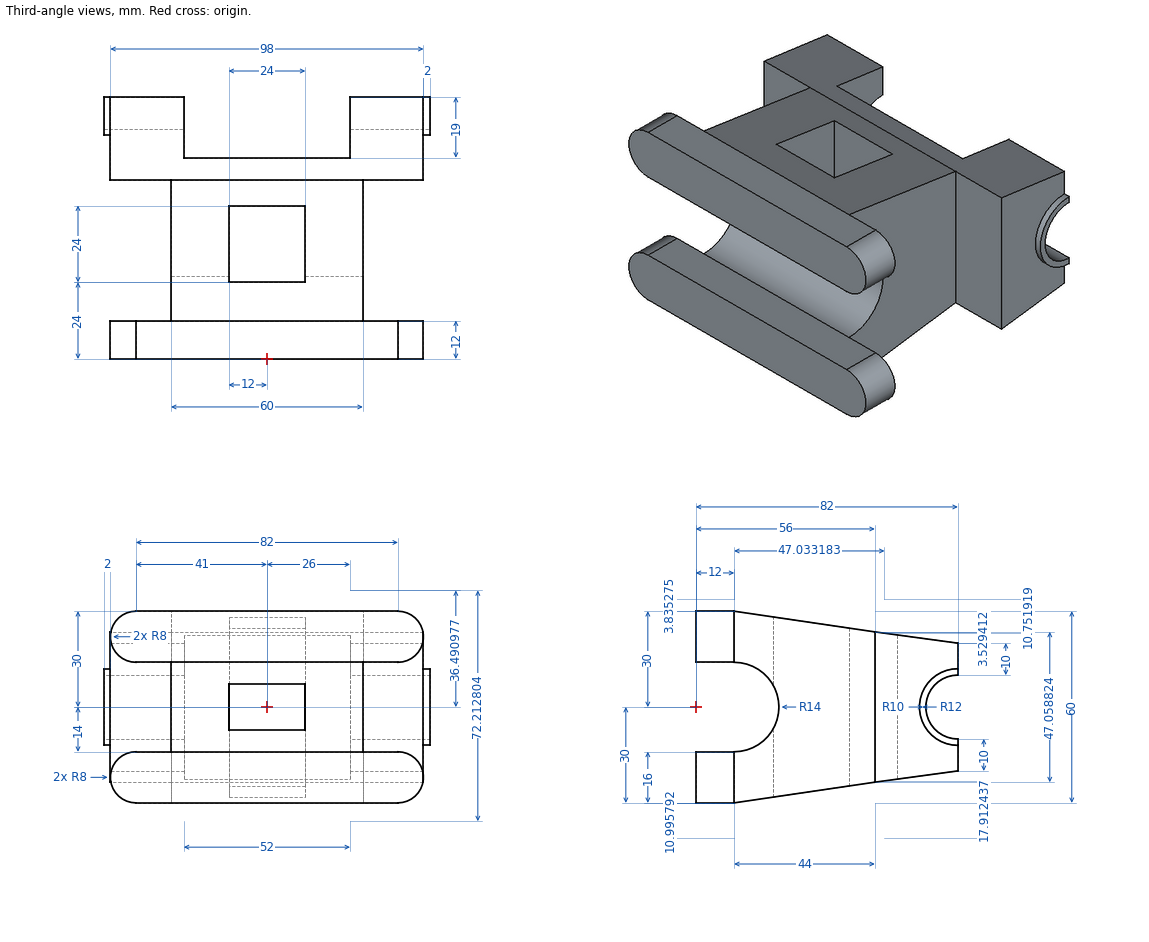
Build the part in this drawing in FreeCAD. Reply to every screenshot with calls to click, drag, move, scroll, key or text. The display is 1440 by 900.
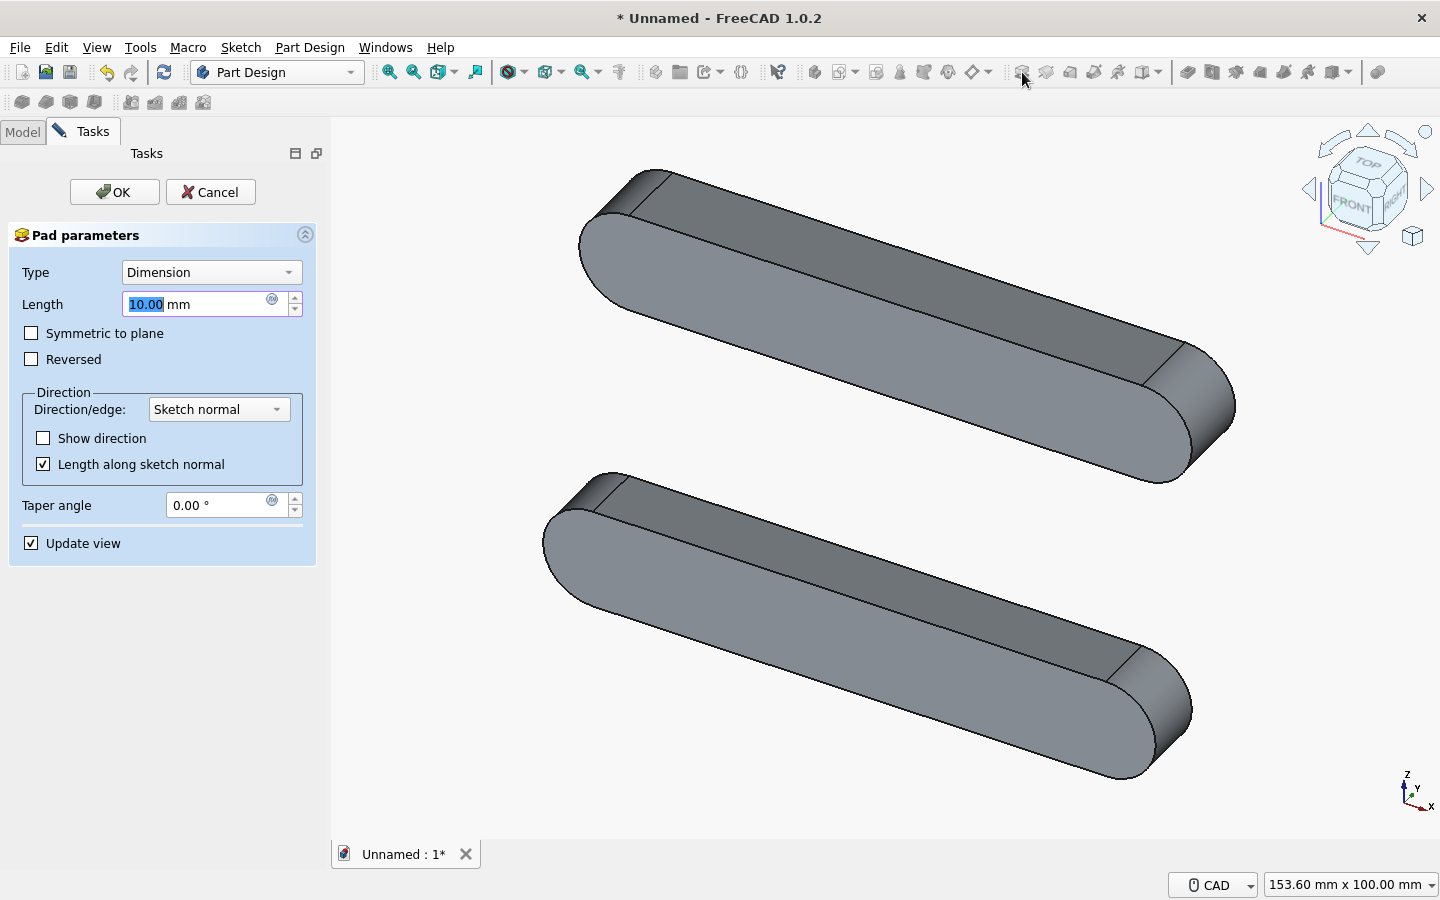
text(12)
key(Tab)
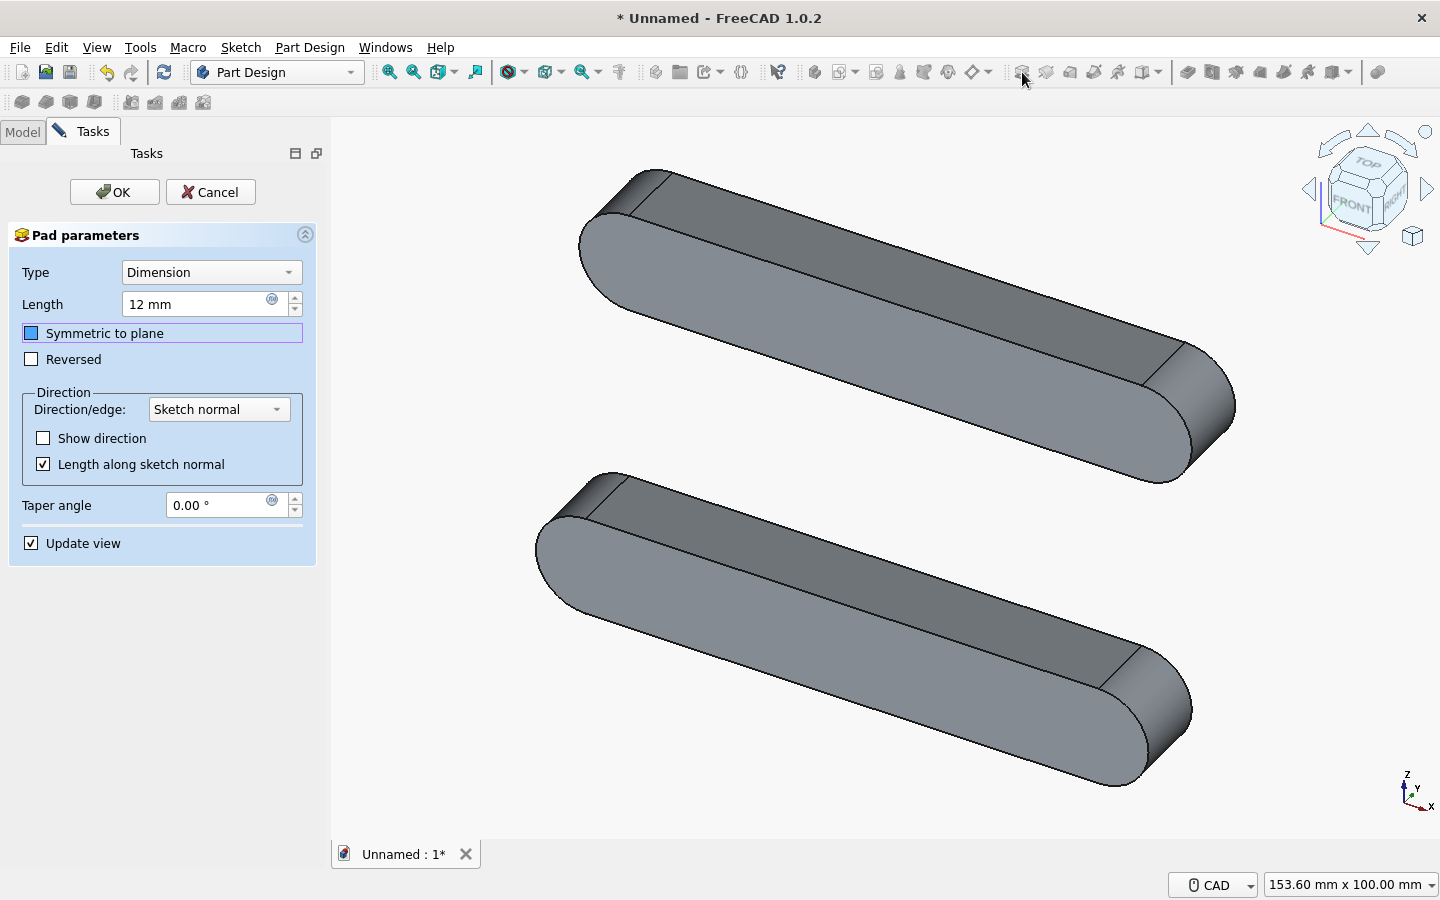
click(30, 359)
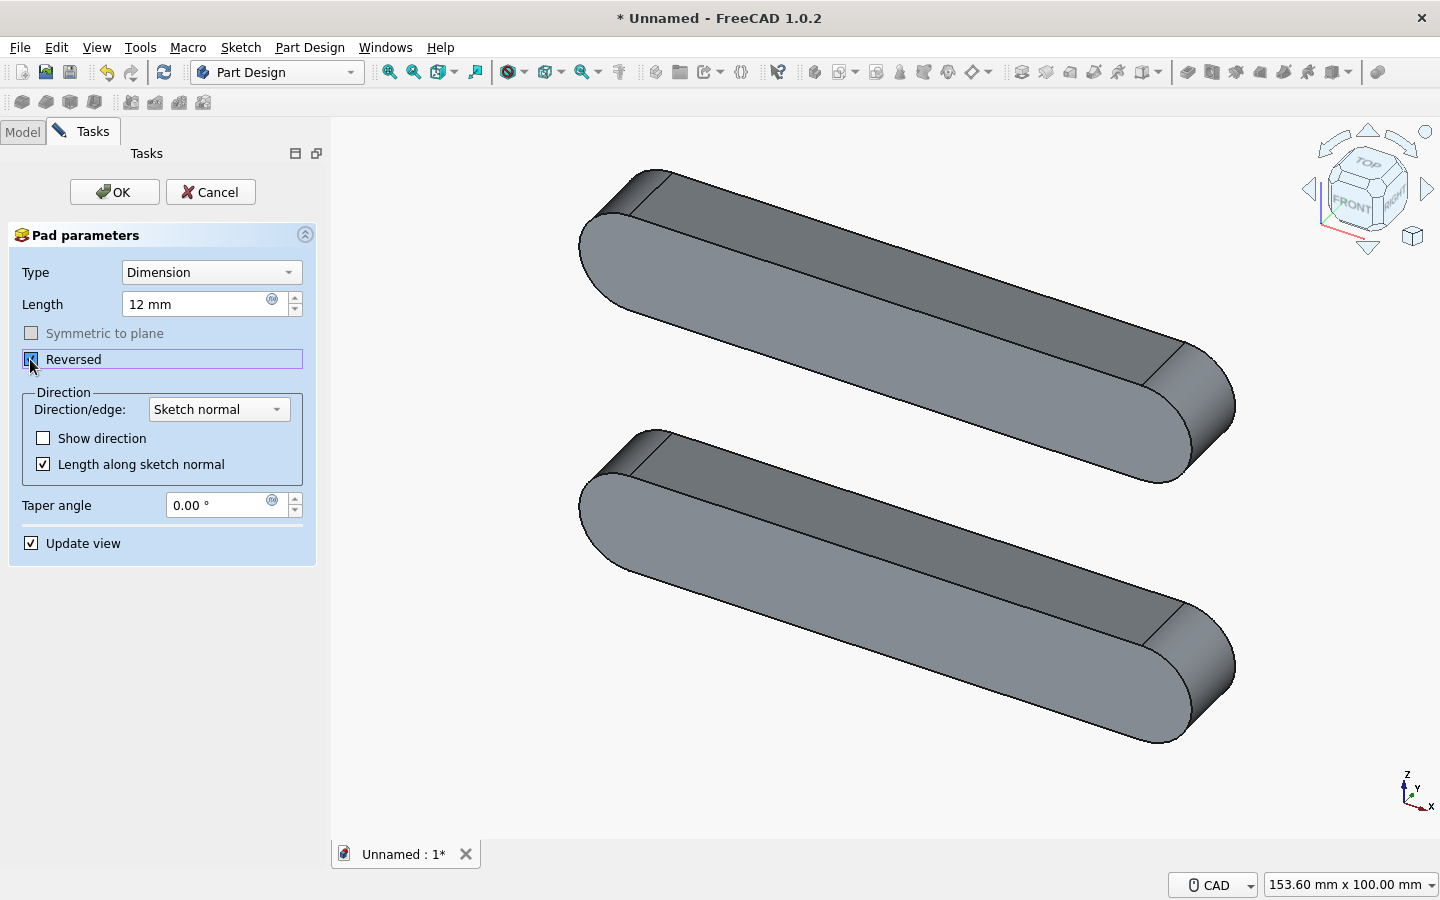
click(115, 192)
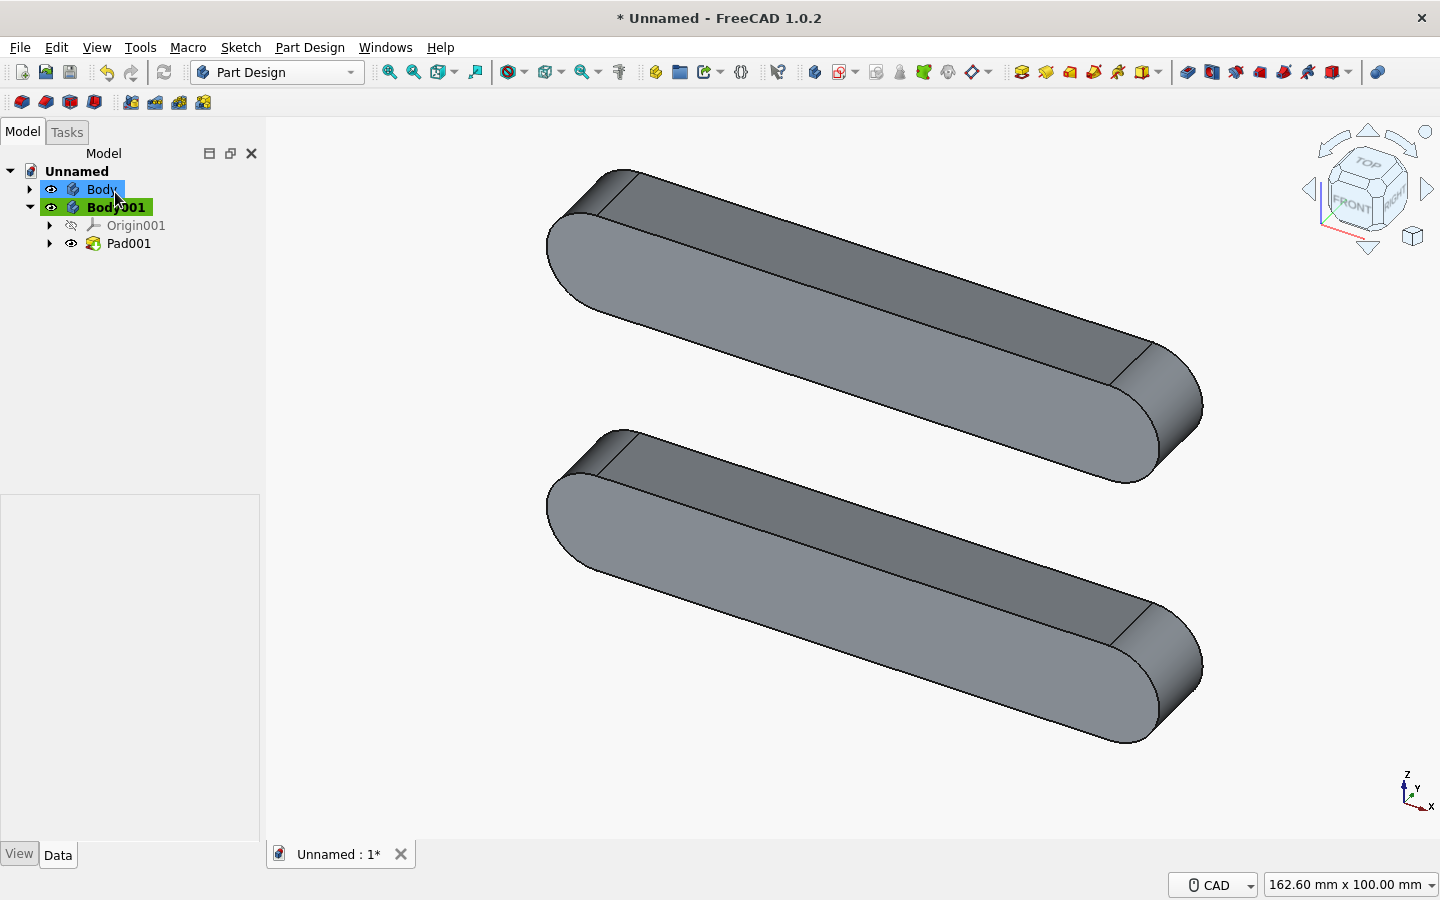
double_click(96, 189)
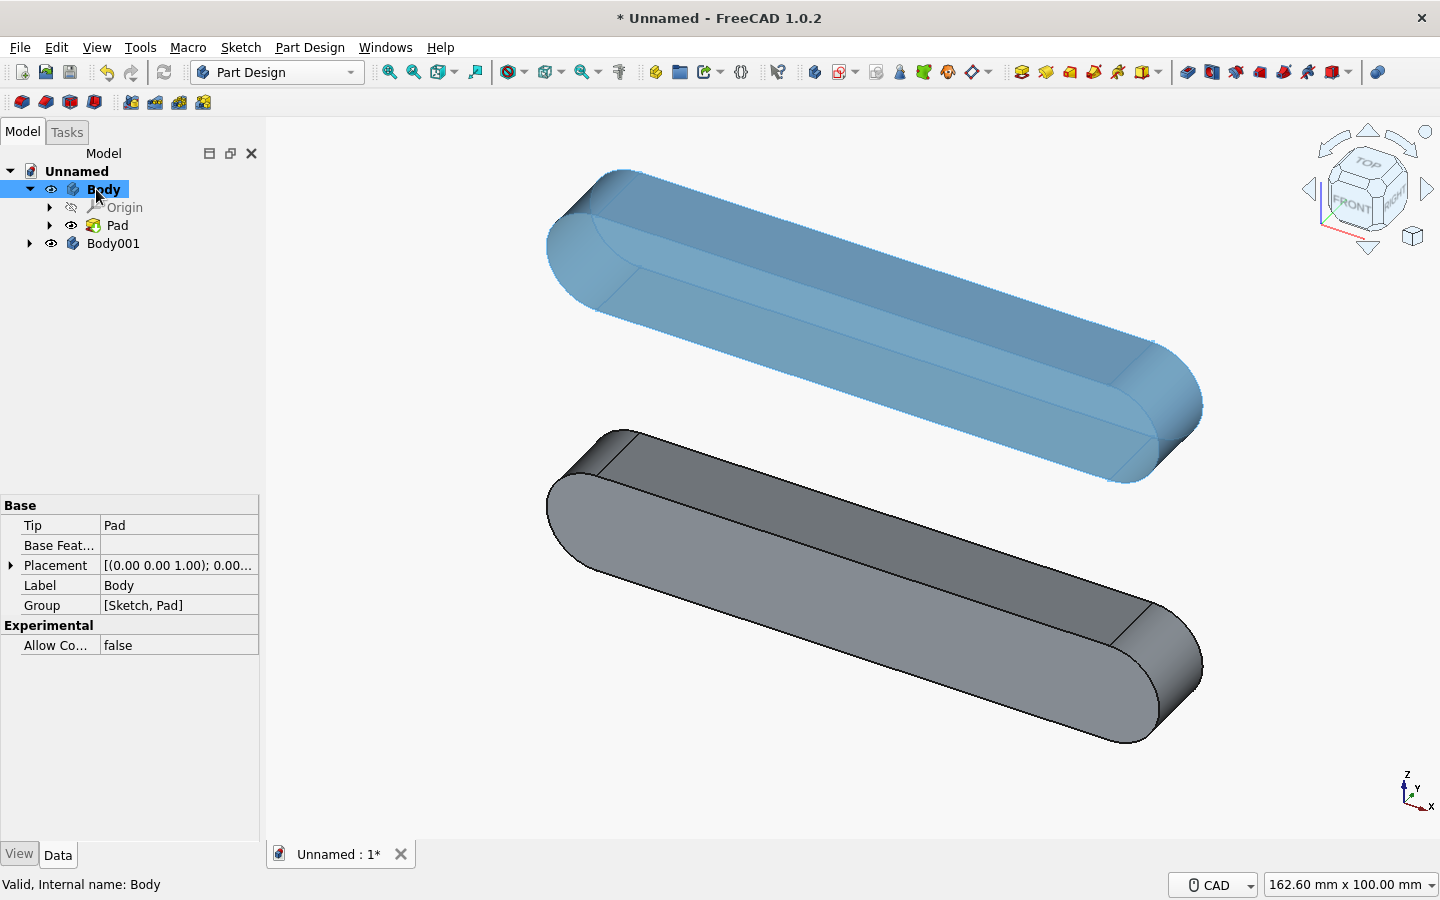
click(96, 189)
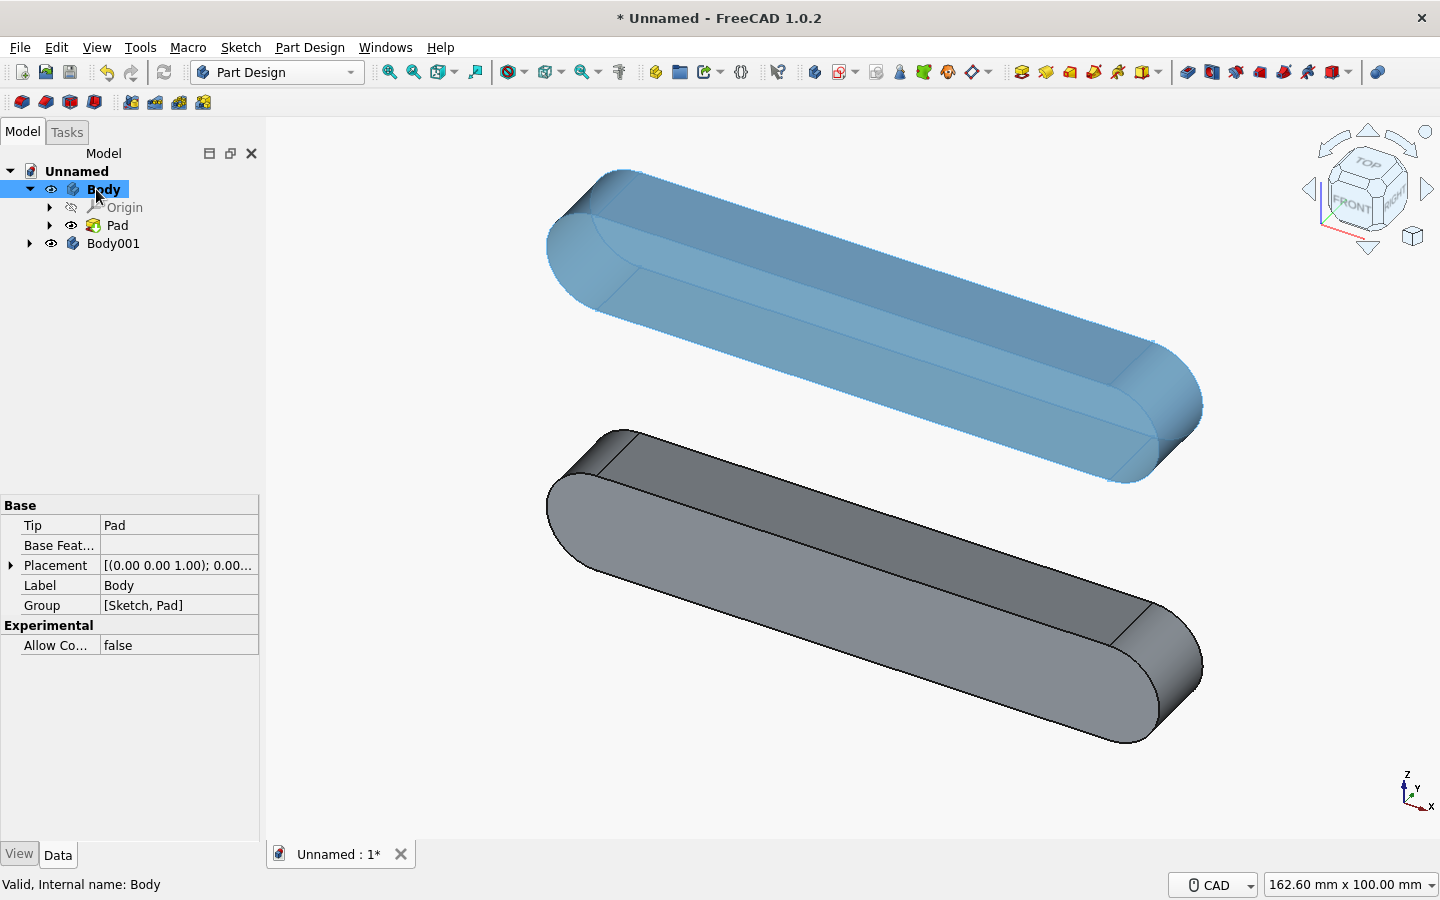
click(146, 645)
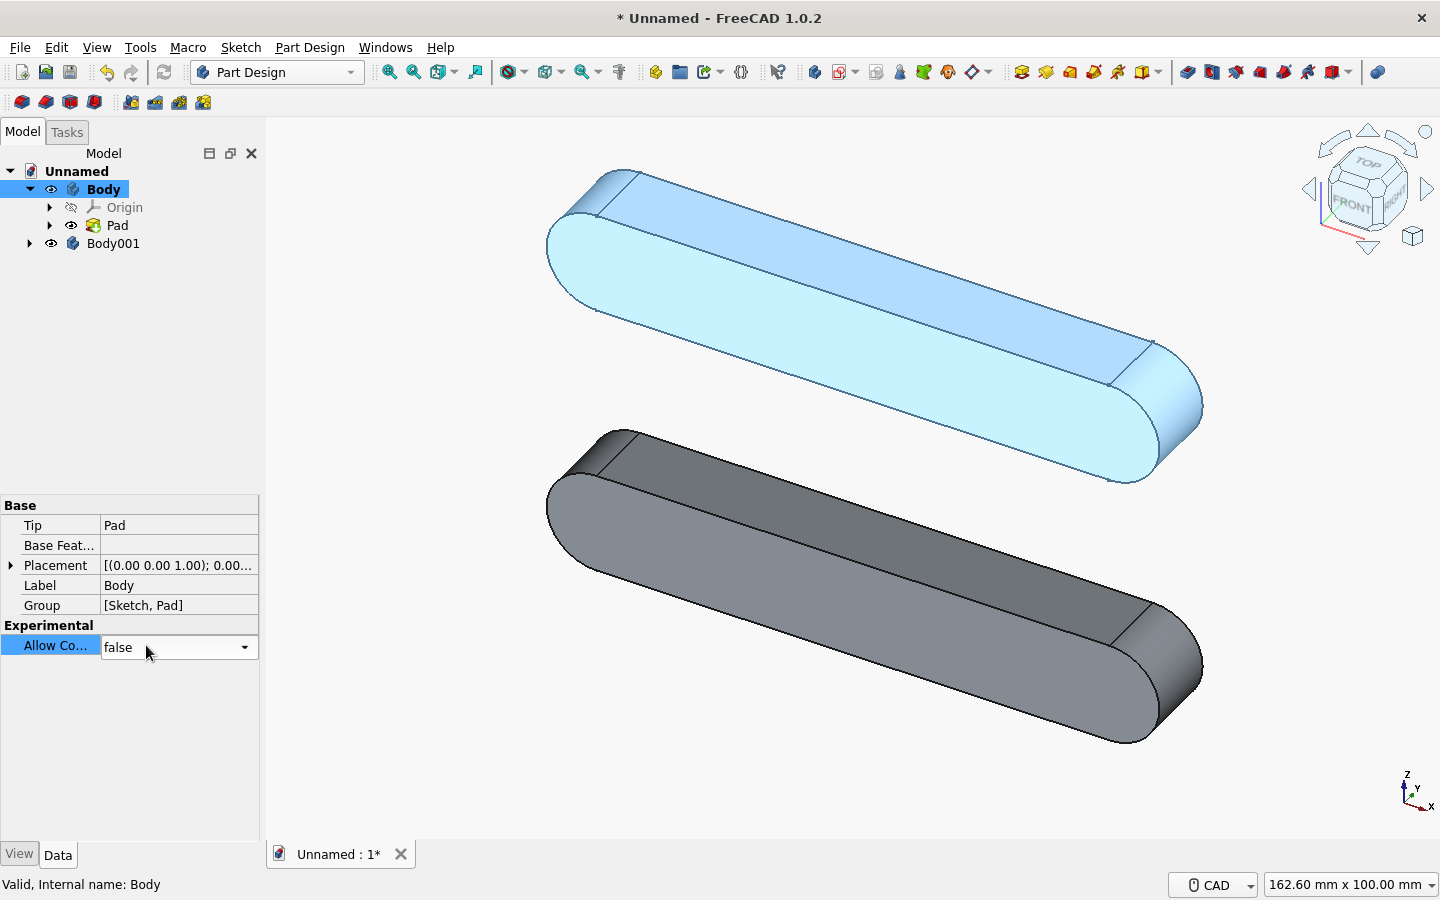
click(146, 645)